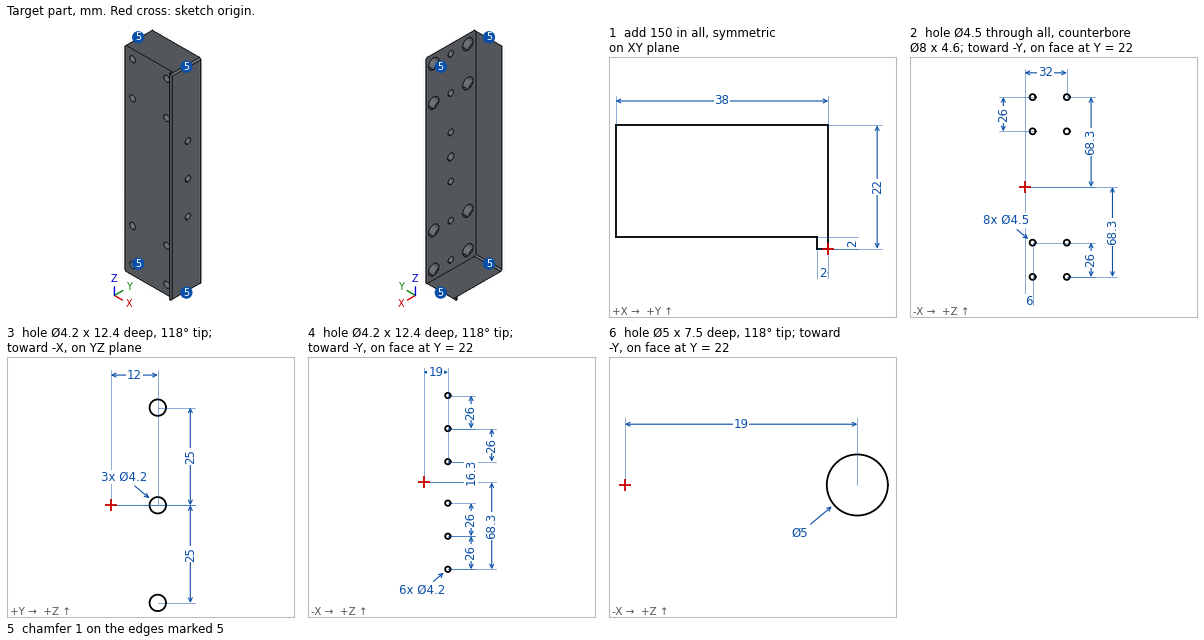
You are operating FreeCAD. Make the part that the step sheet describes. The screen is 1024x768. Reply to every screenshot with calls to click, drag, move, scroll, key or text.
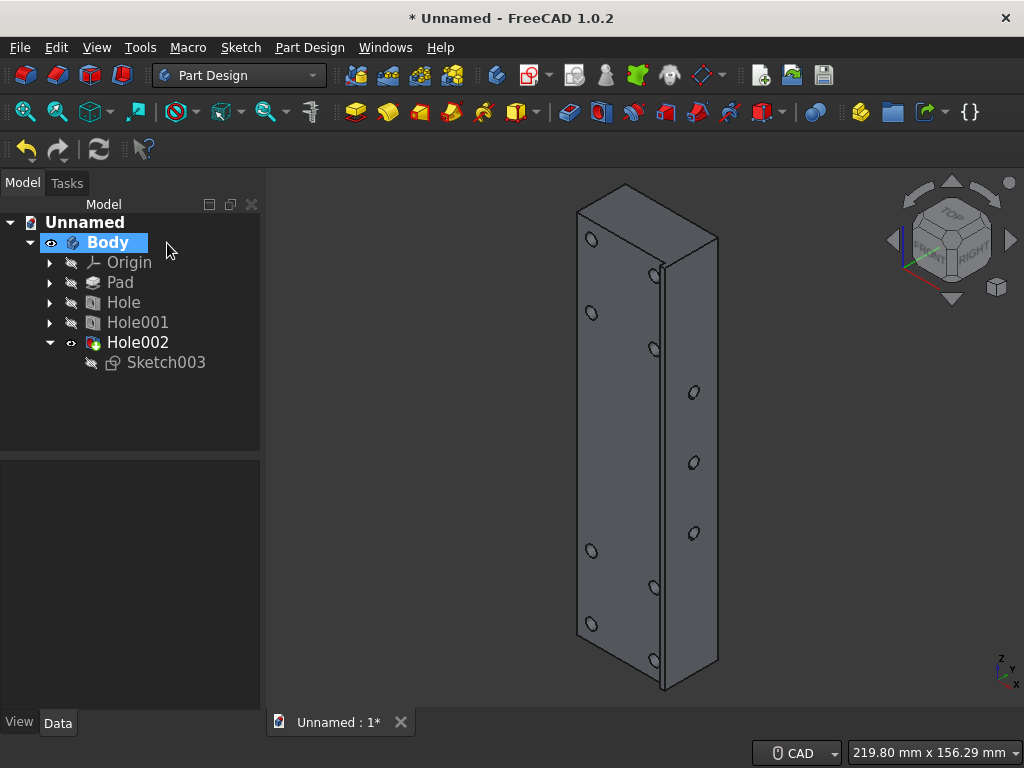
click(691, 252)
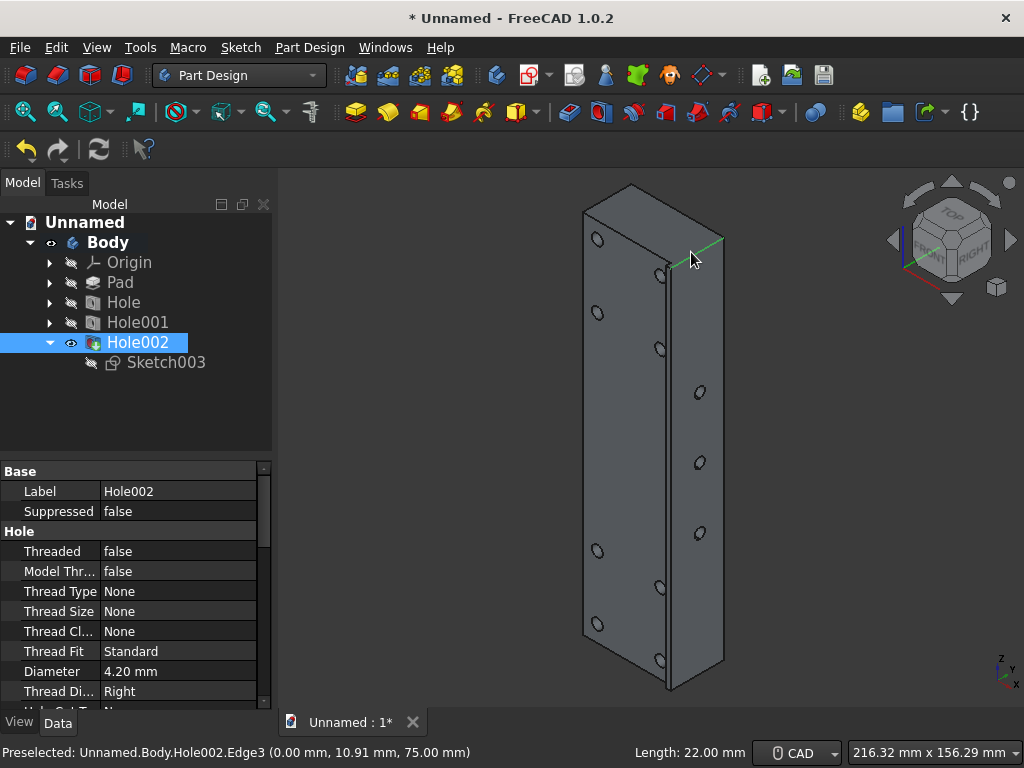
key(2)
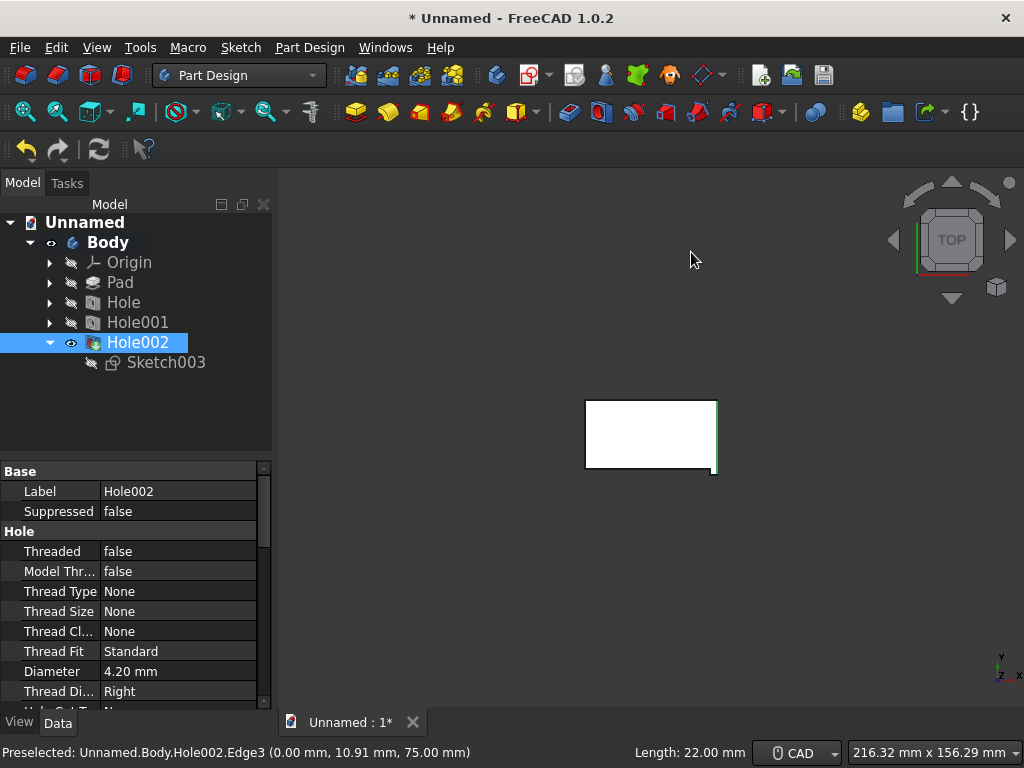
key(v)
key(f)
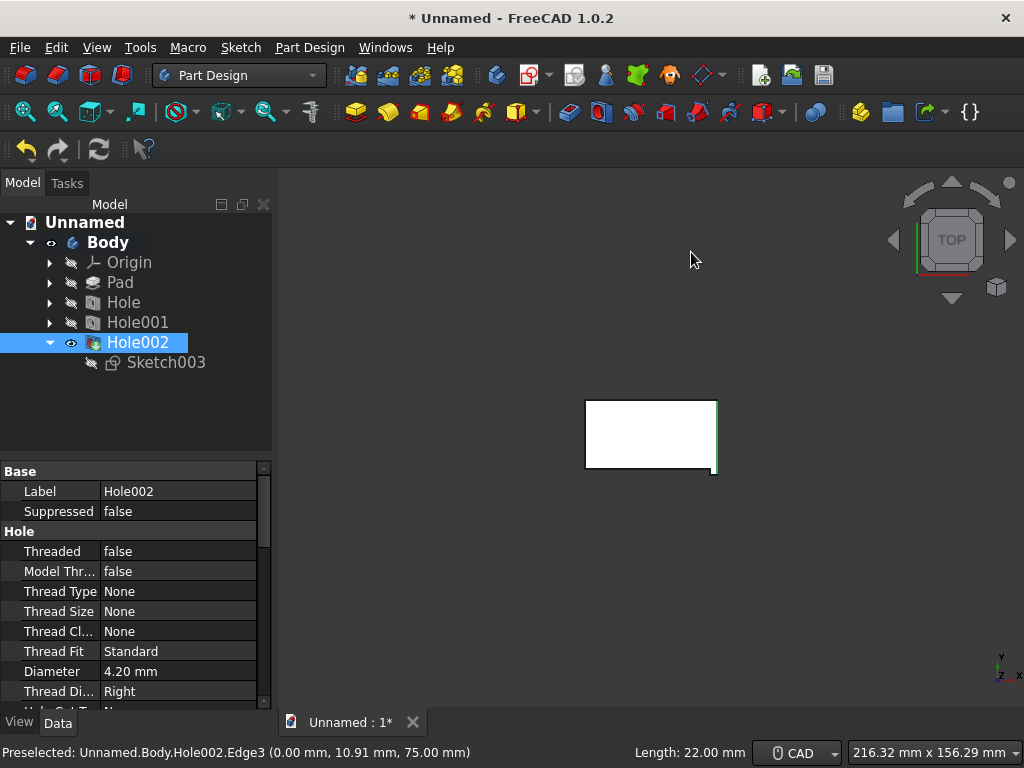
click(585, 433, ctrl)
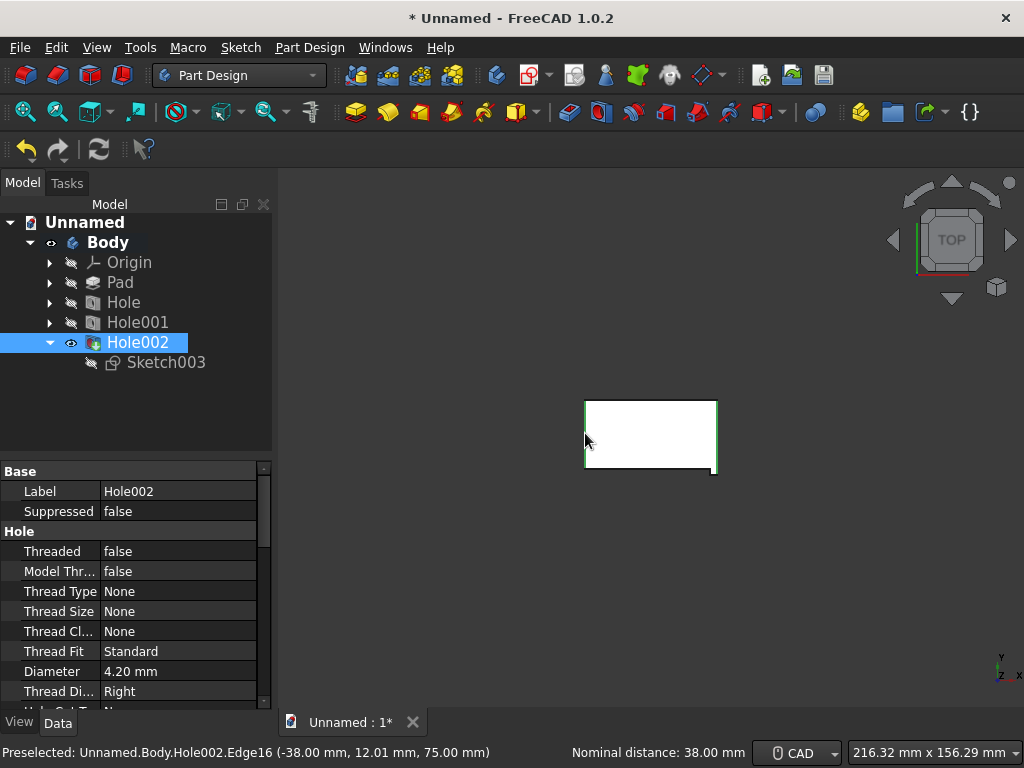
key(1)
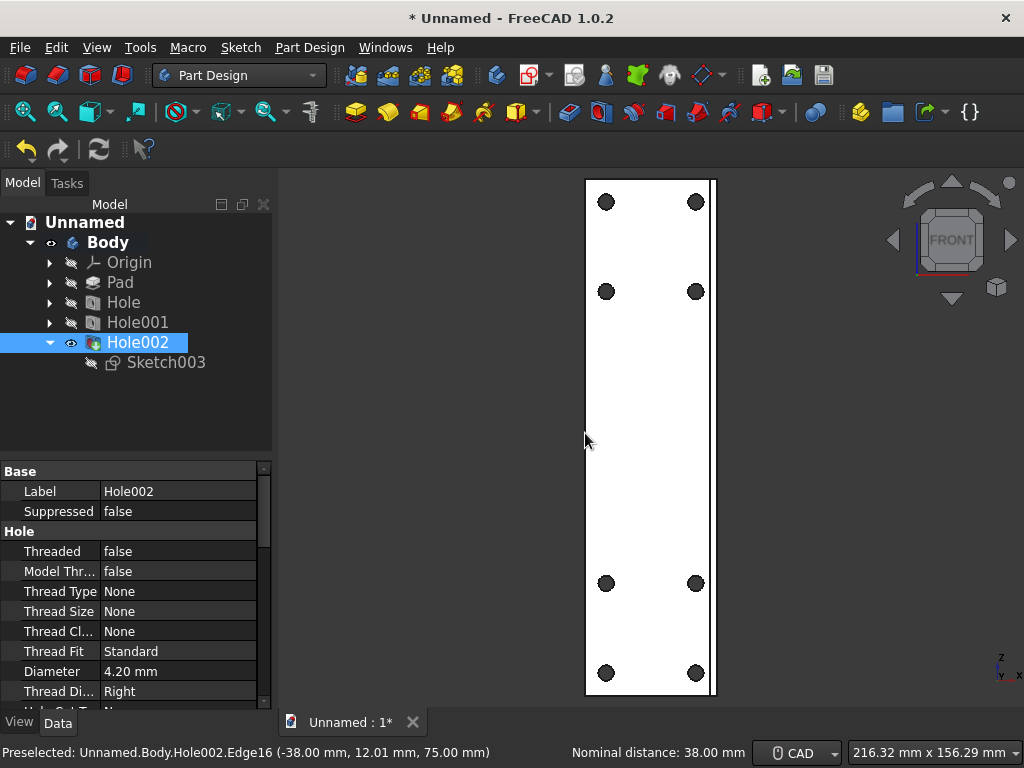
key(3)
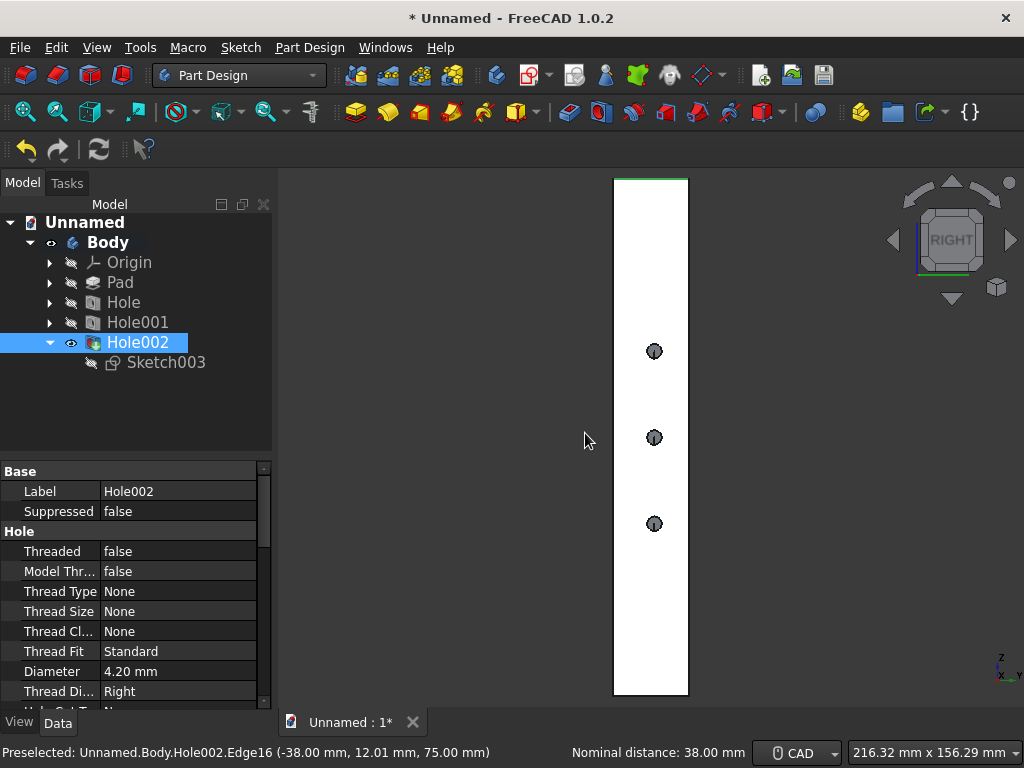
key(5)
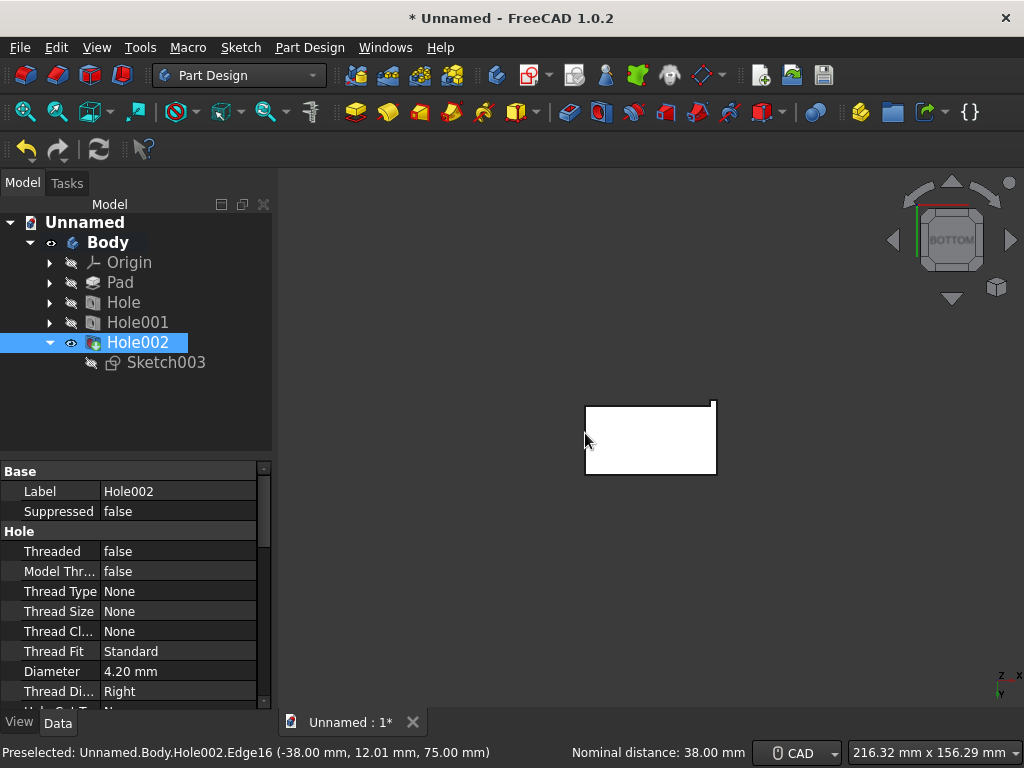
click(26, 112)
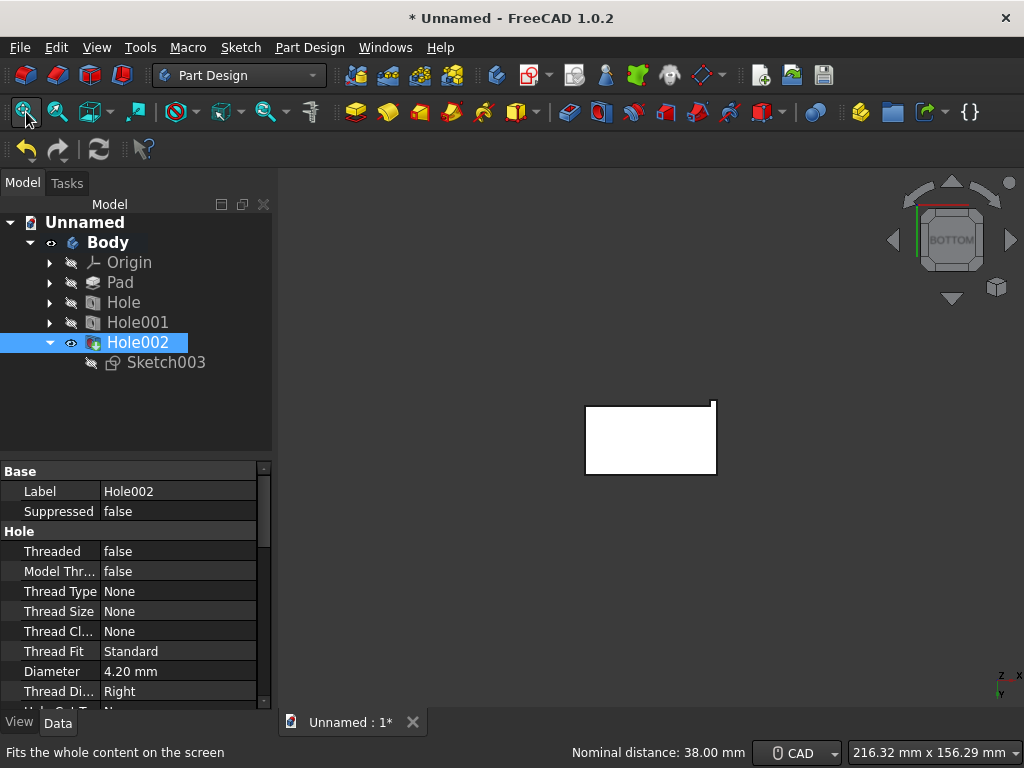
click(585, 440, ctrl)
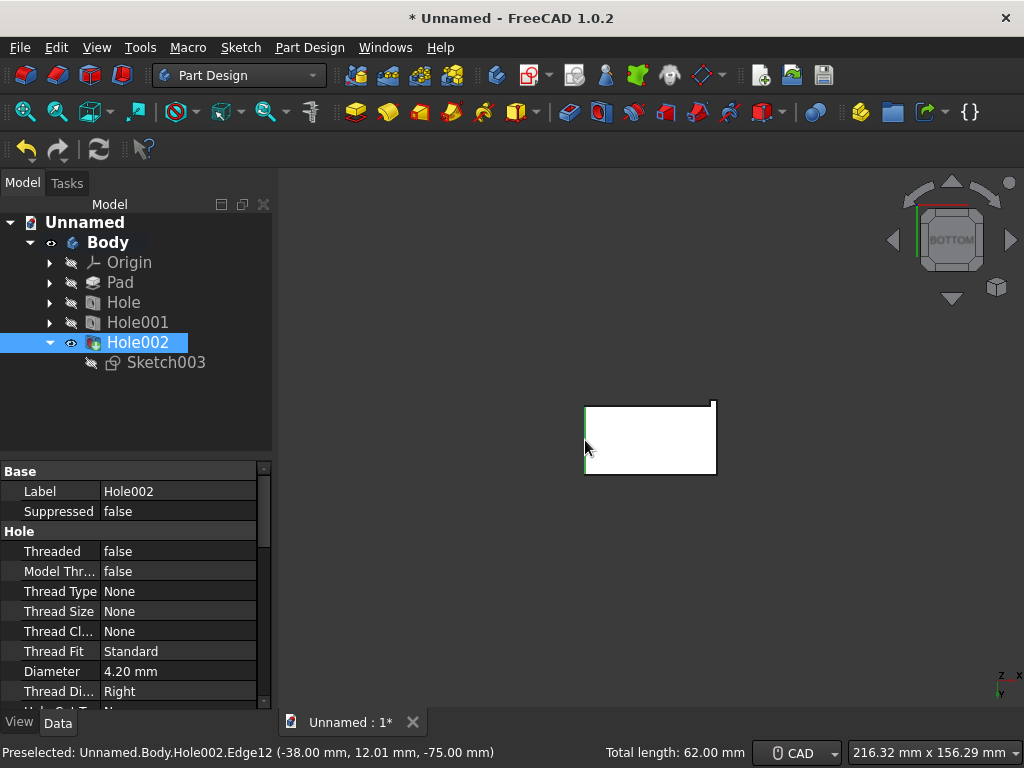
click(717, 436, ctrl)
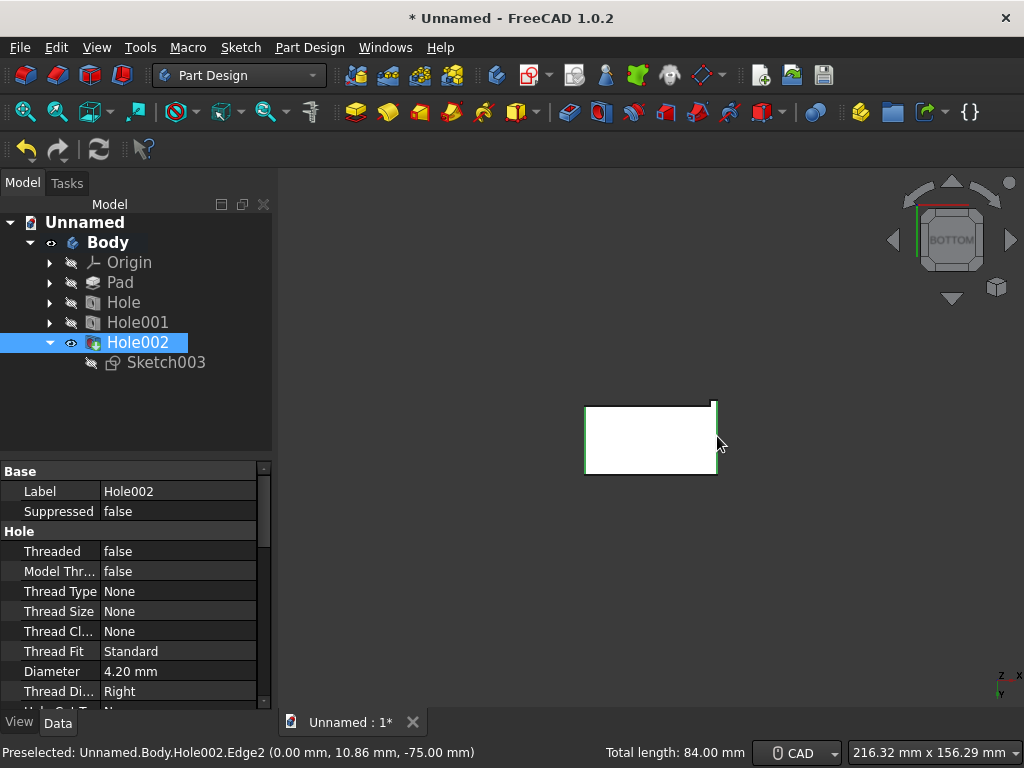
click(58, 76)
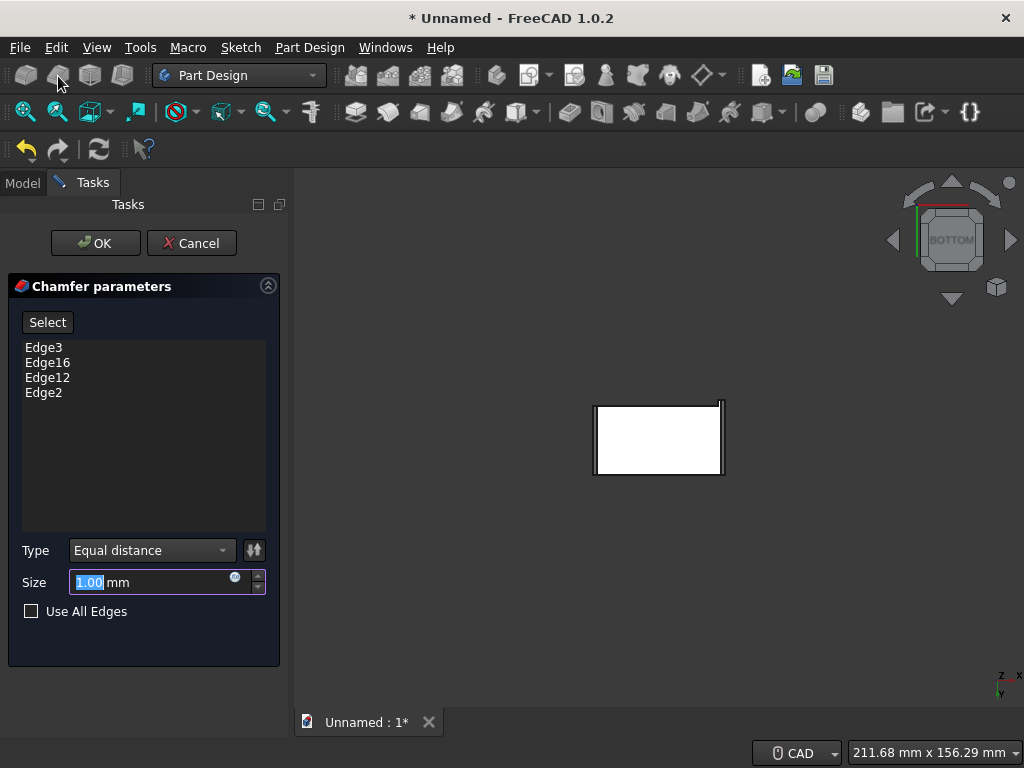
text(1)
key(Tab)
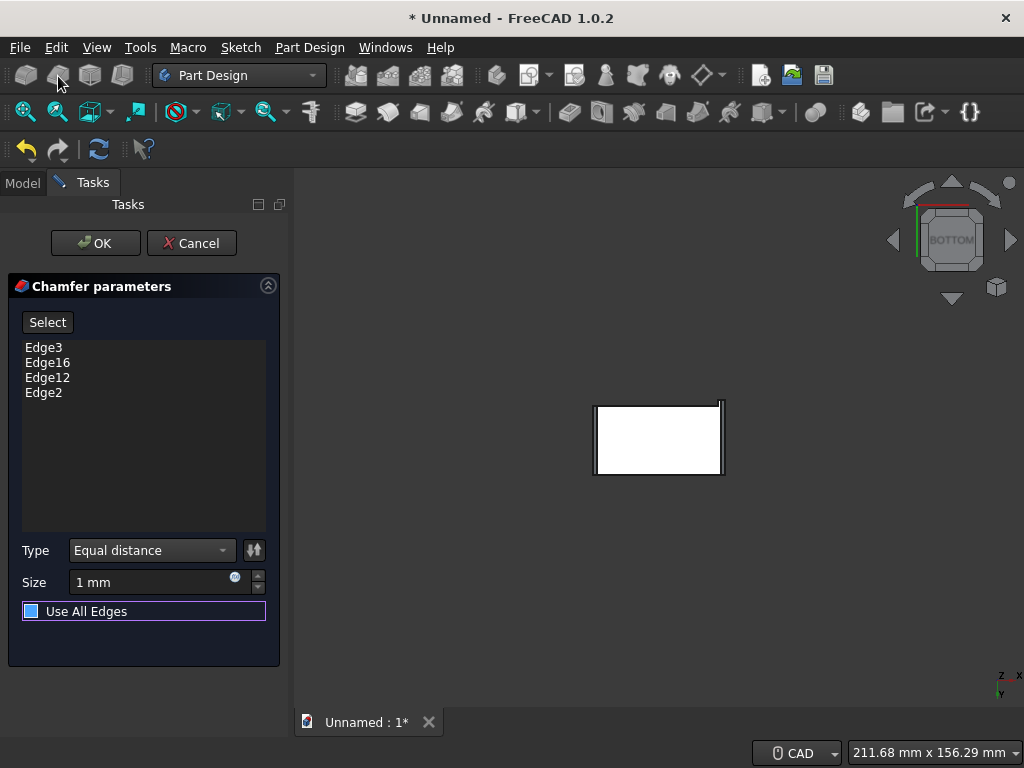
click(96, 243)